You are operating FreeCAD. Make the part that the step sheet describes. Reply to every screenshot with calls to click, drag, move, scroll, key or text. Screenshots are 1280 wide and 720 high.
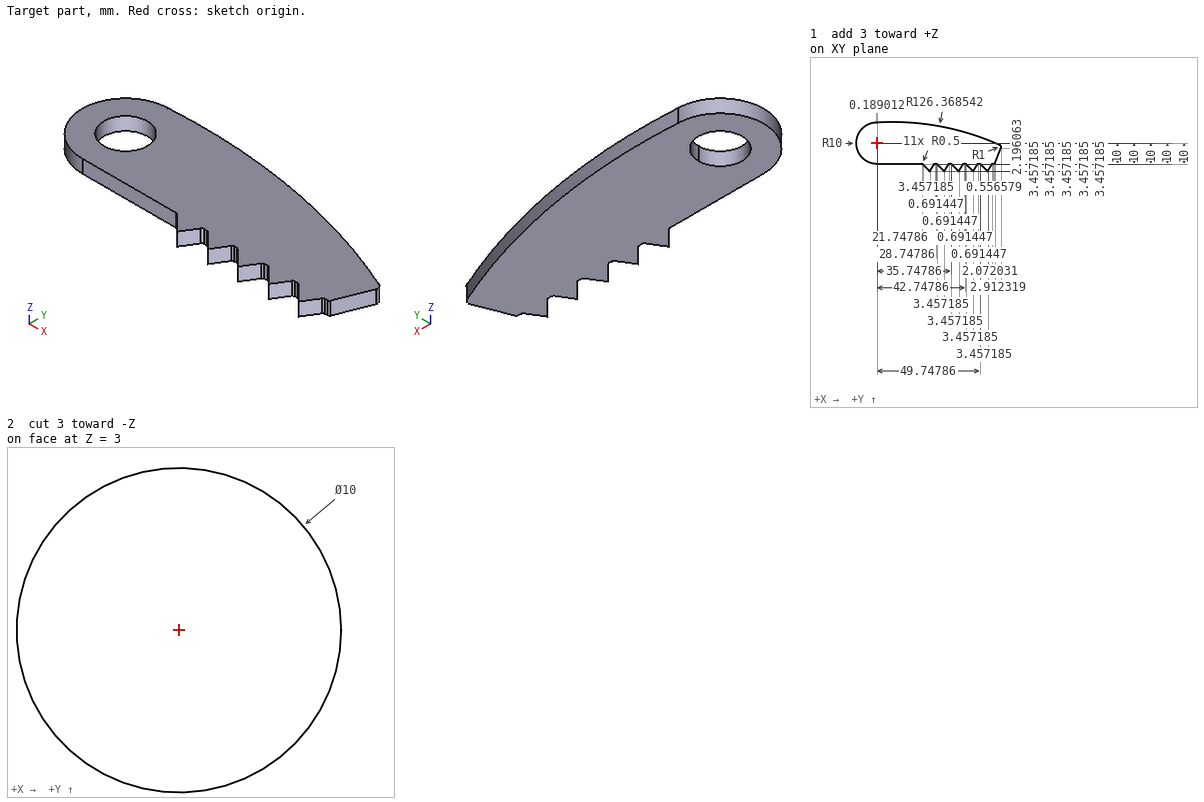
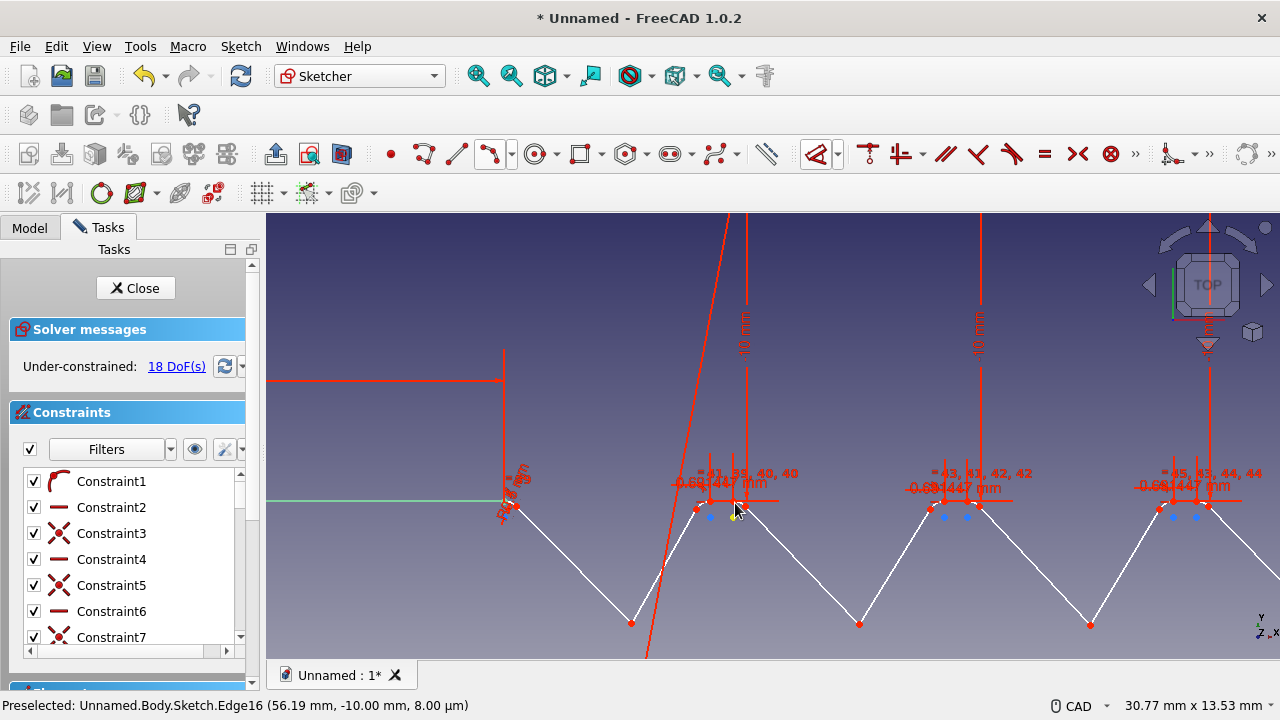
click(733, 501)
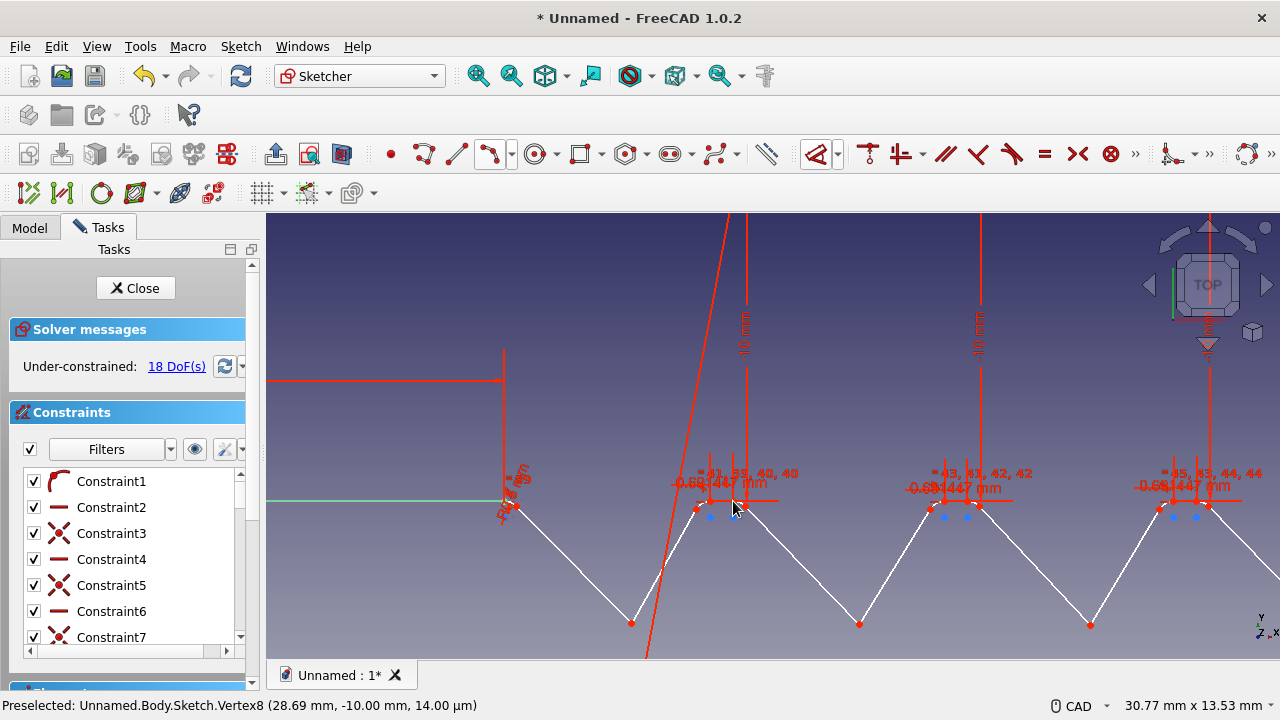
click(838, 154)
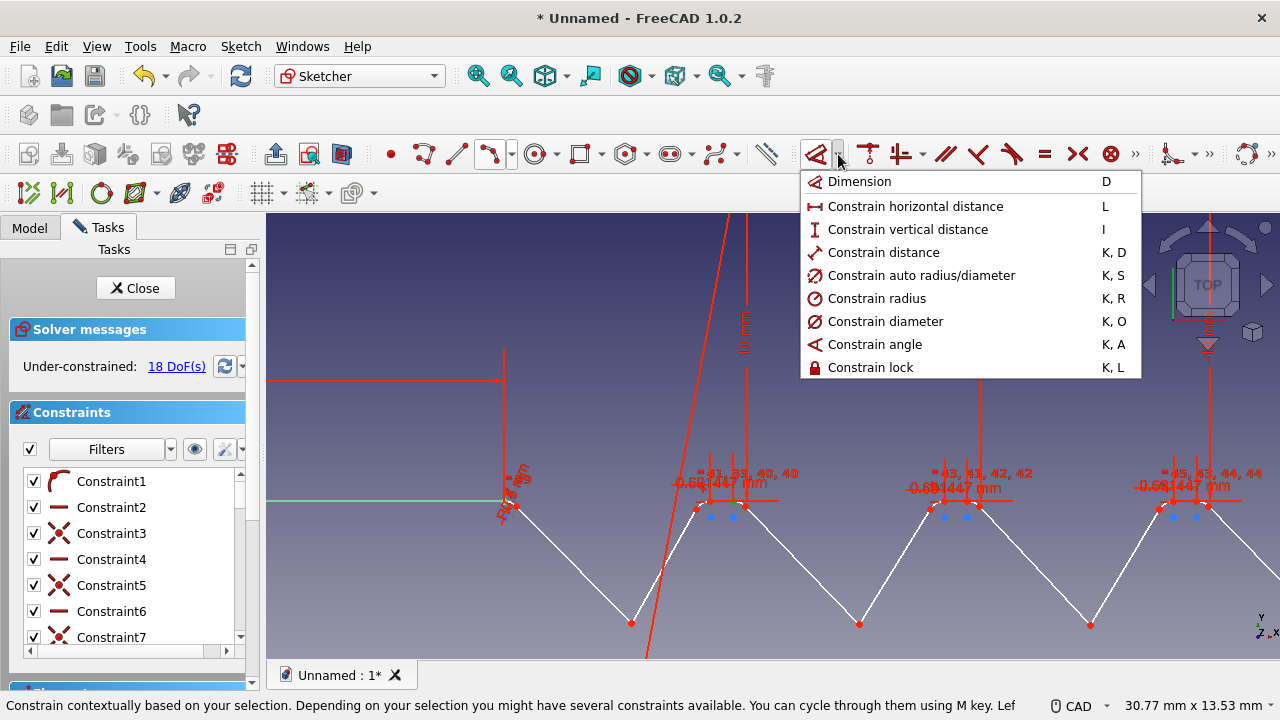
click(971, 206)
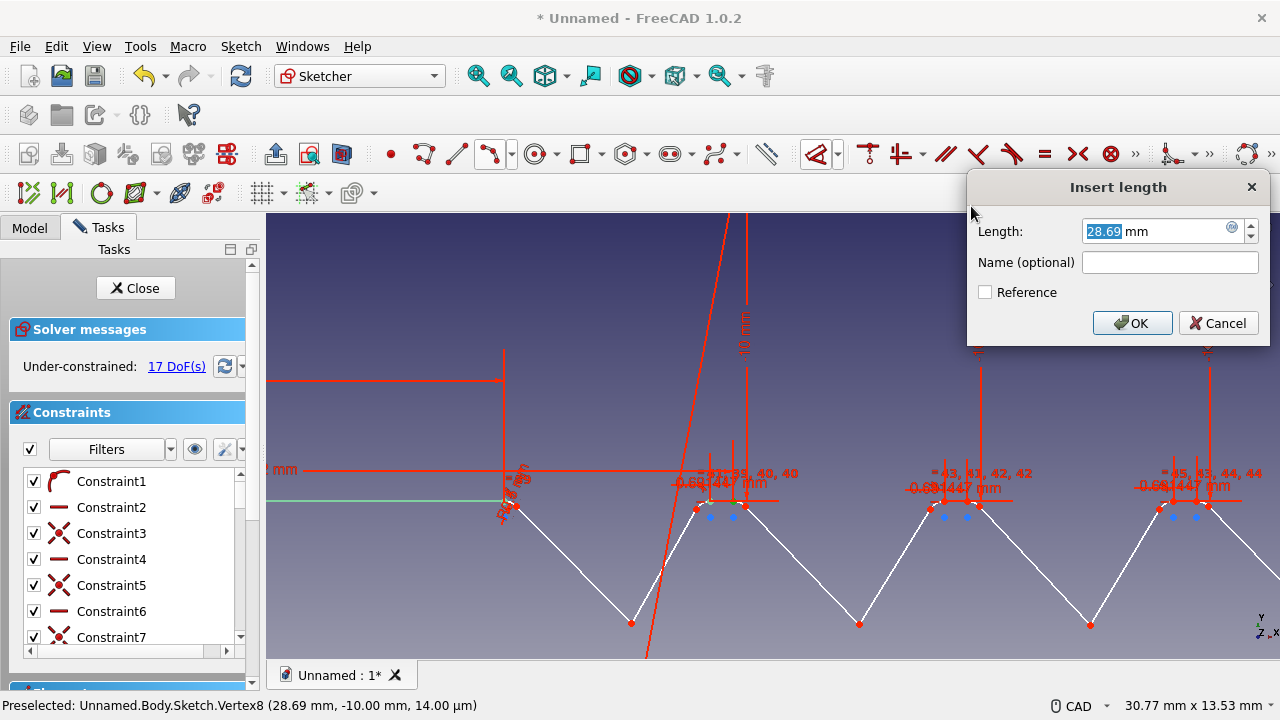
text(28.74786)
key(Return)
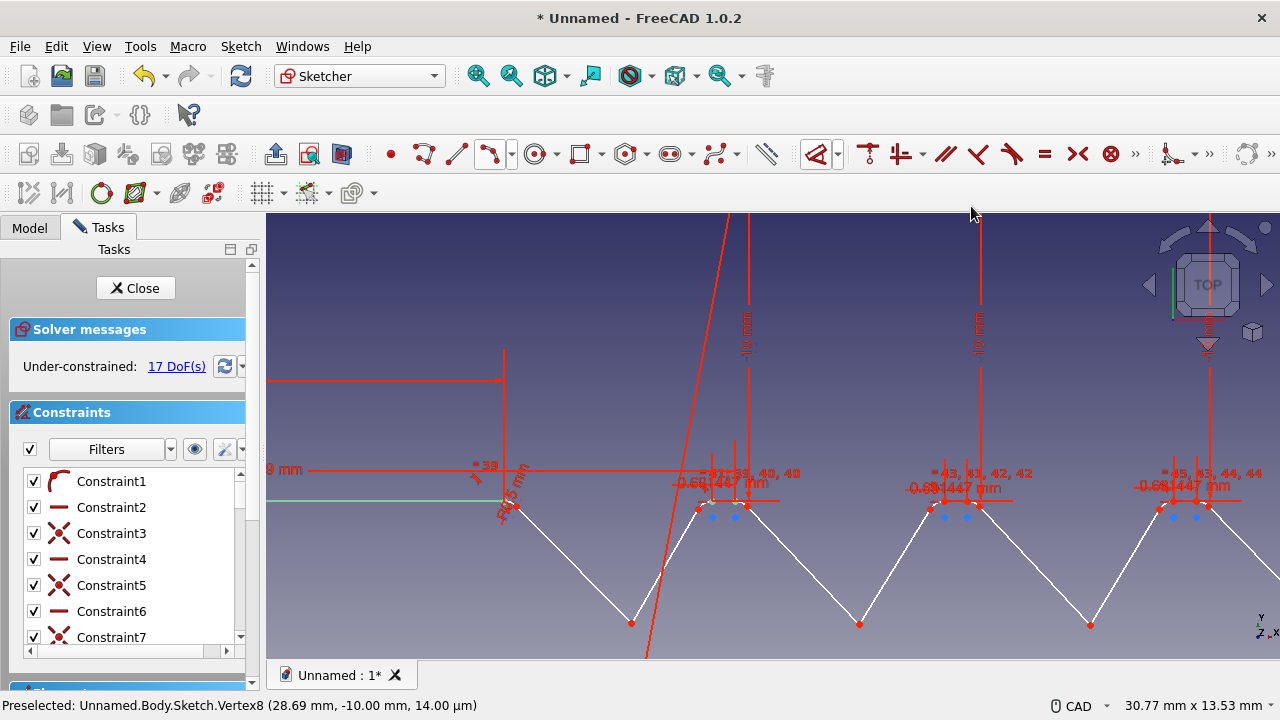
click(967, 501)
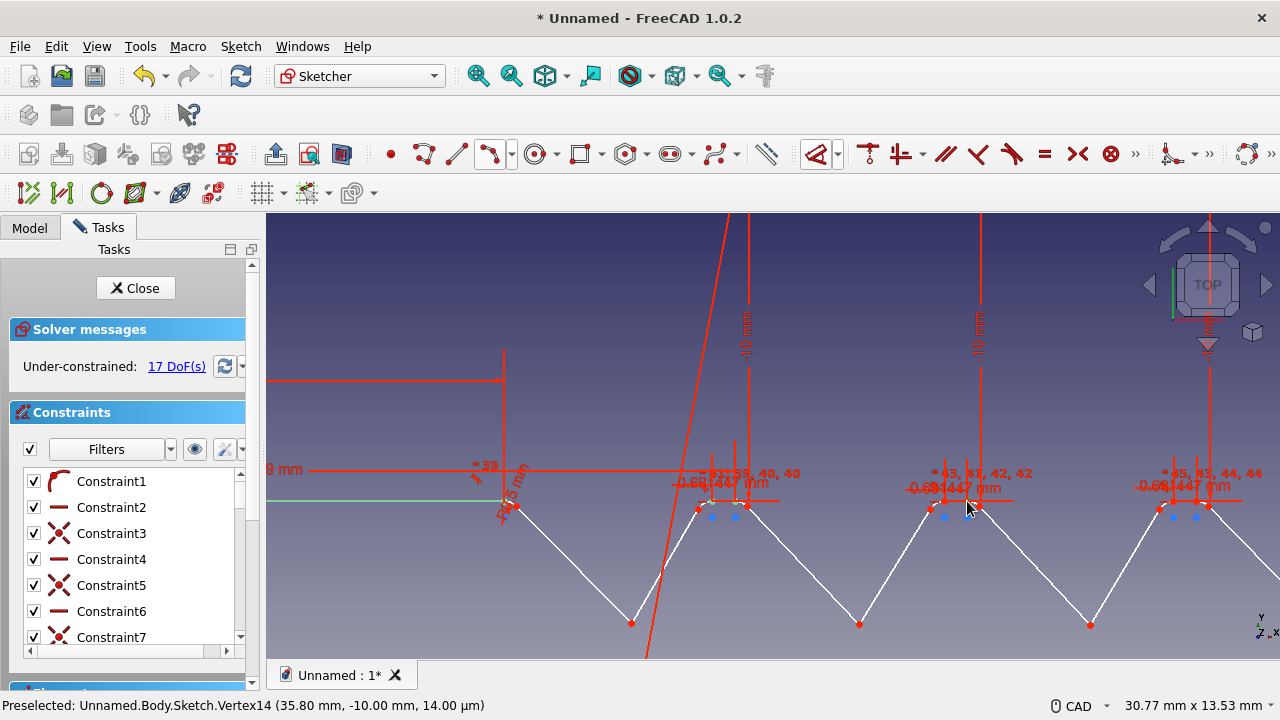
key(l)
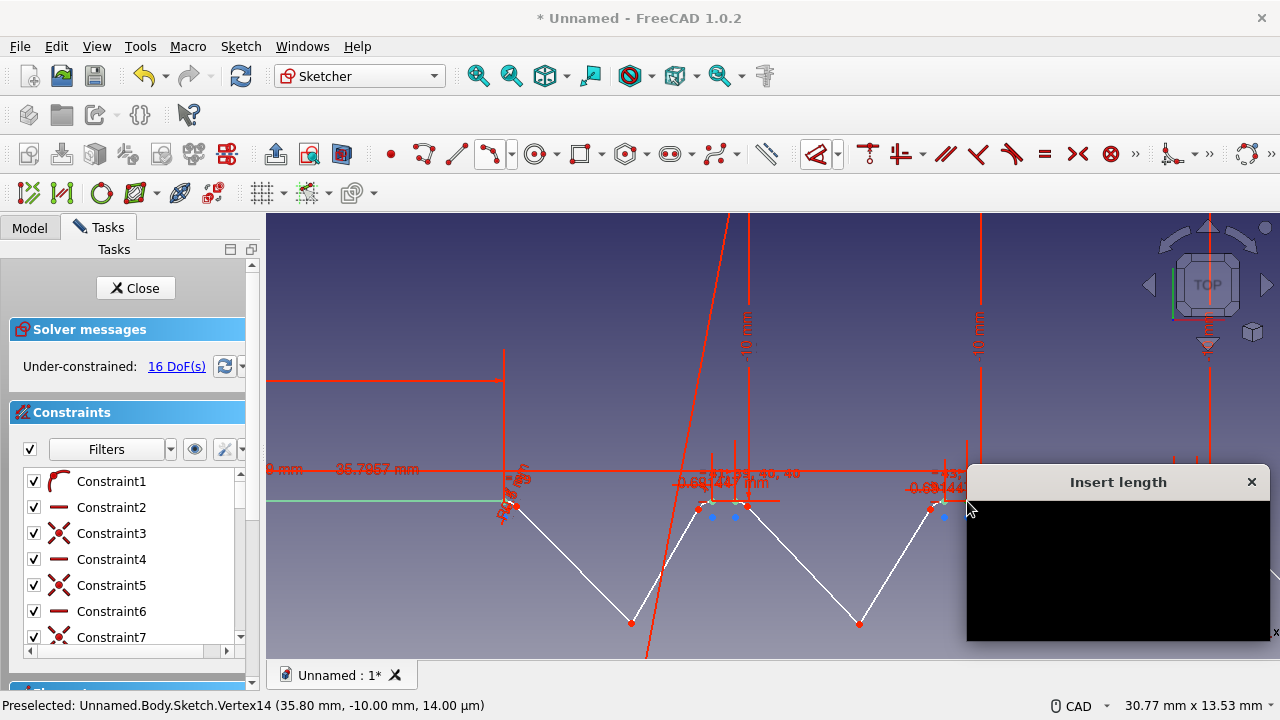
text(35.74786)
key(Return)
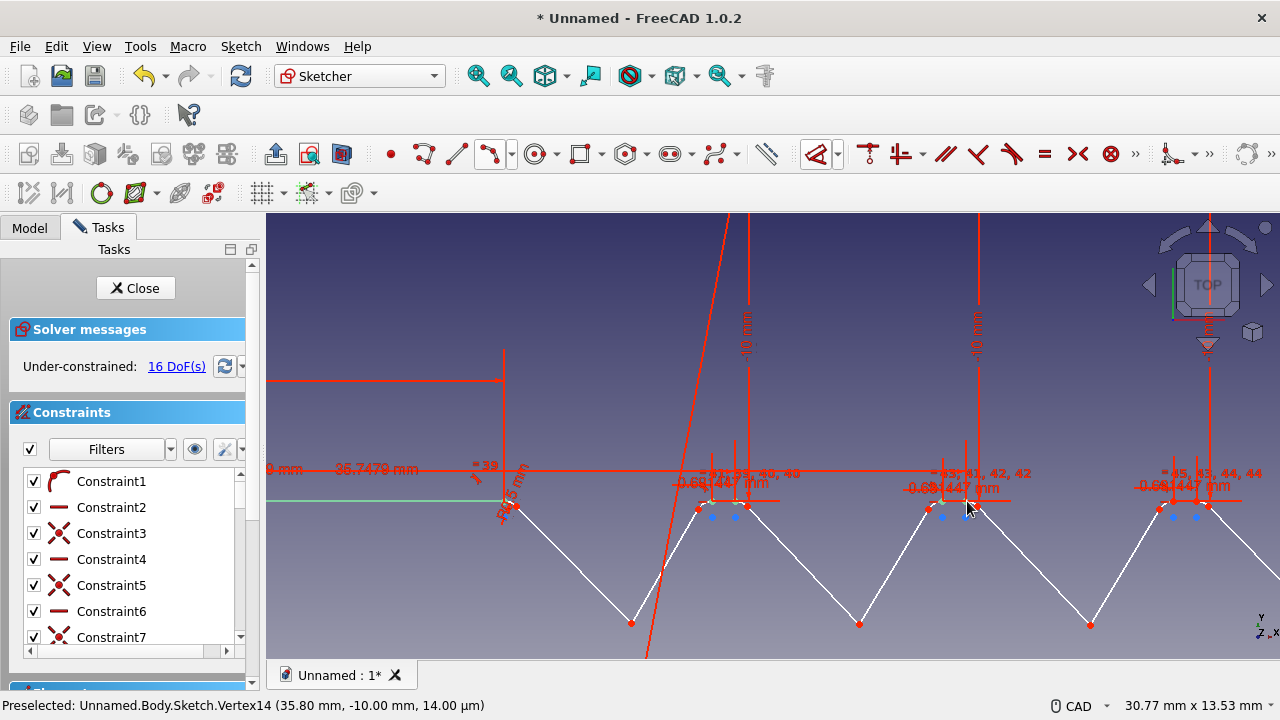
scroll(735, 503, down, 7)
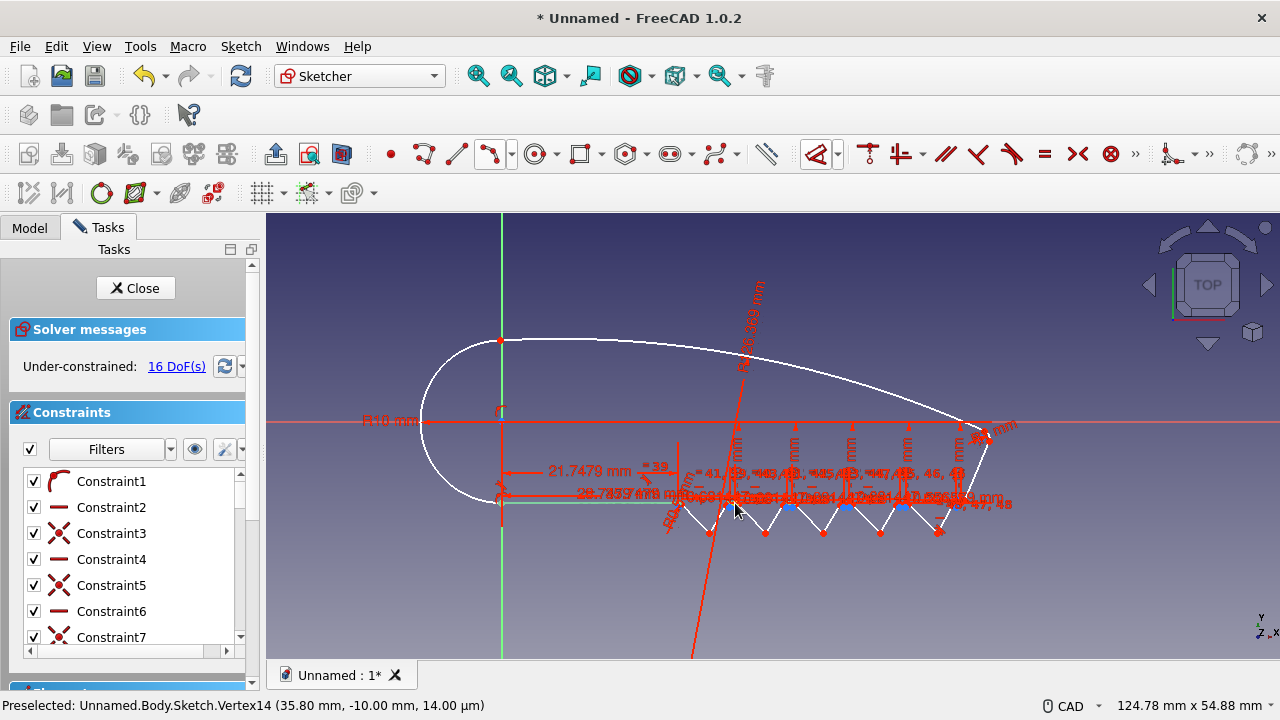
scroll(849, 503, up, 7)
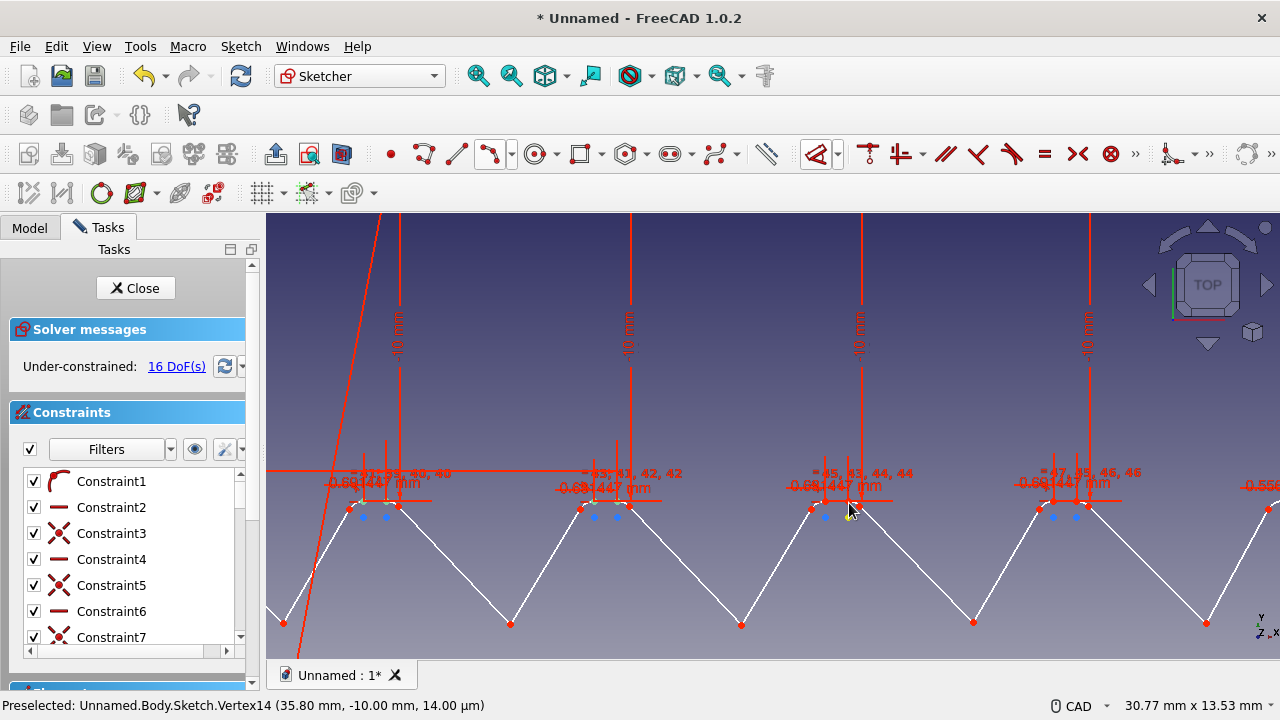
click(848, 501)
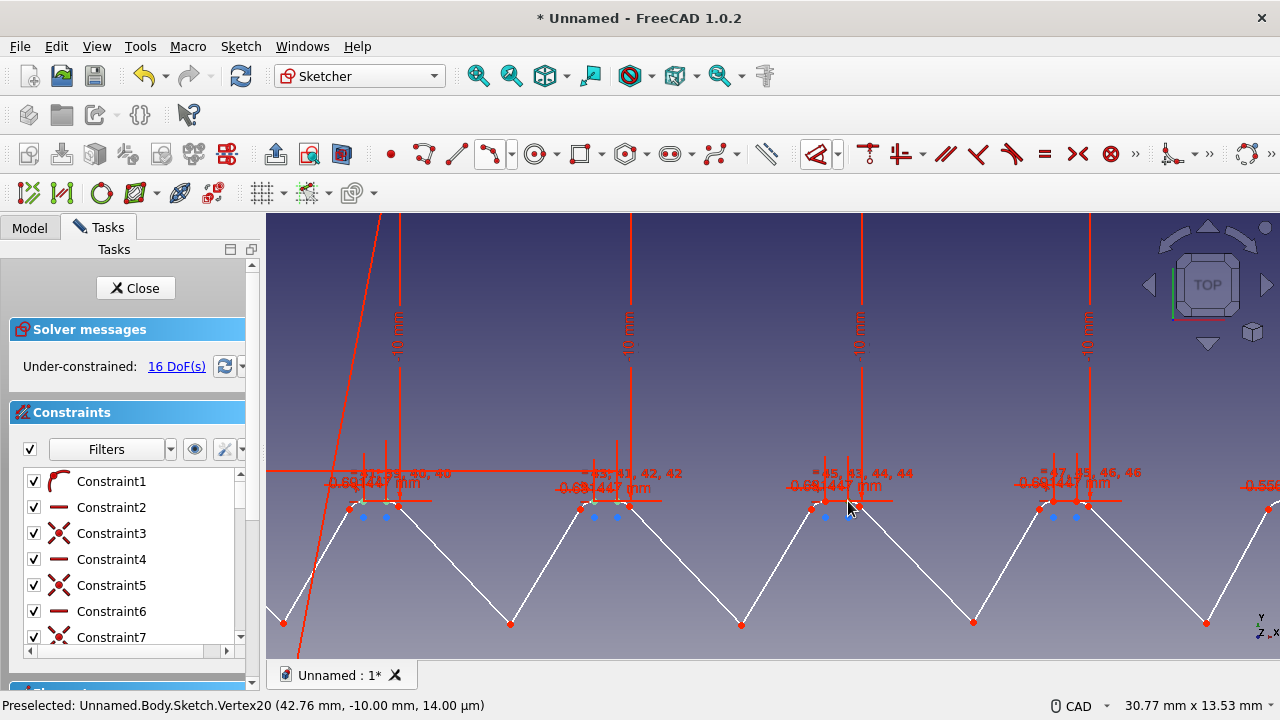
key(l)